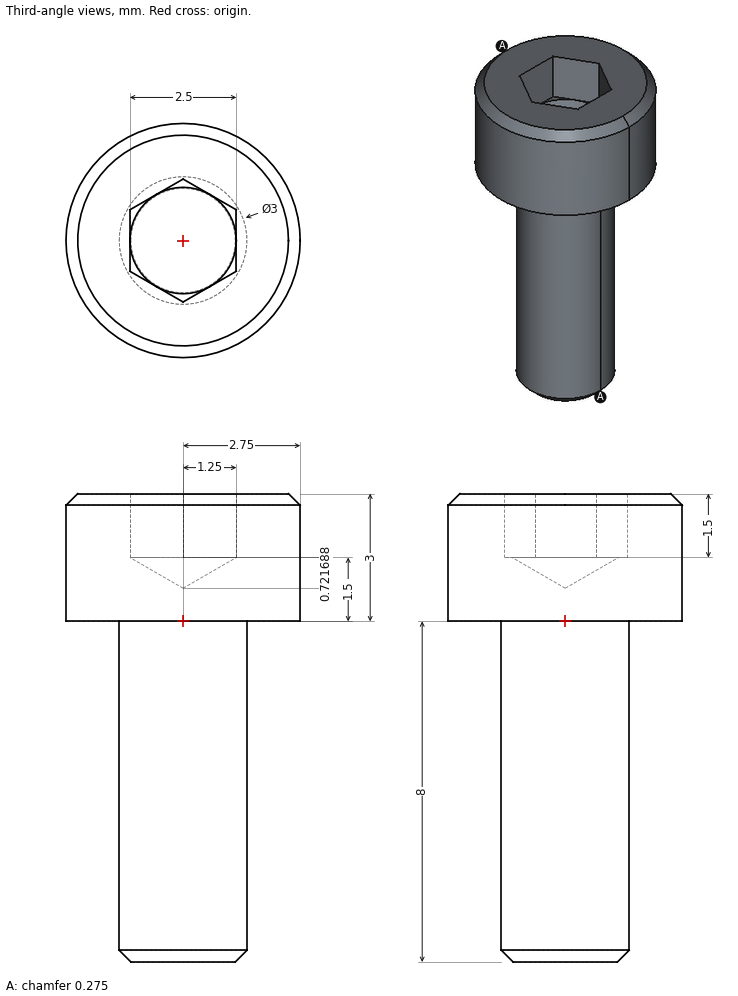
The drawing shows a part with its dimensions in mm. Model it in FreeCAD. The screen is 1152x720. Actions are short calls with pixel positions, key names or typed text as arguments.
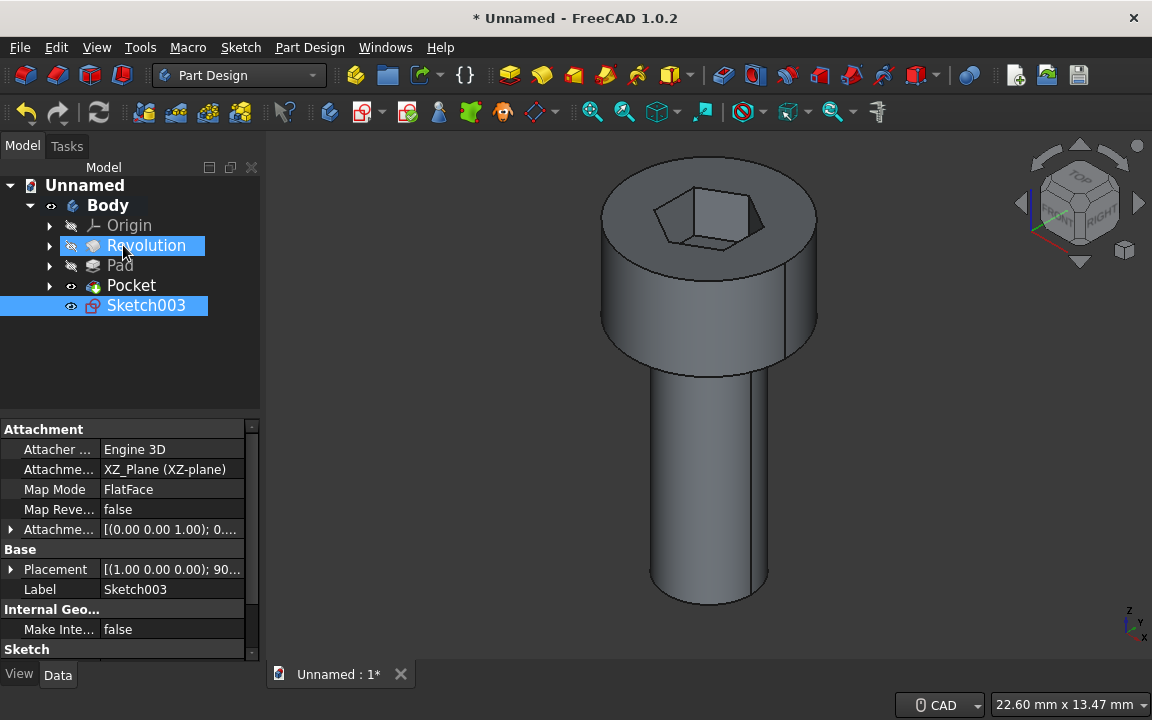
click(788, 76)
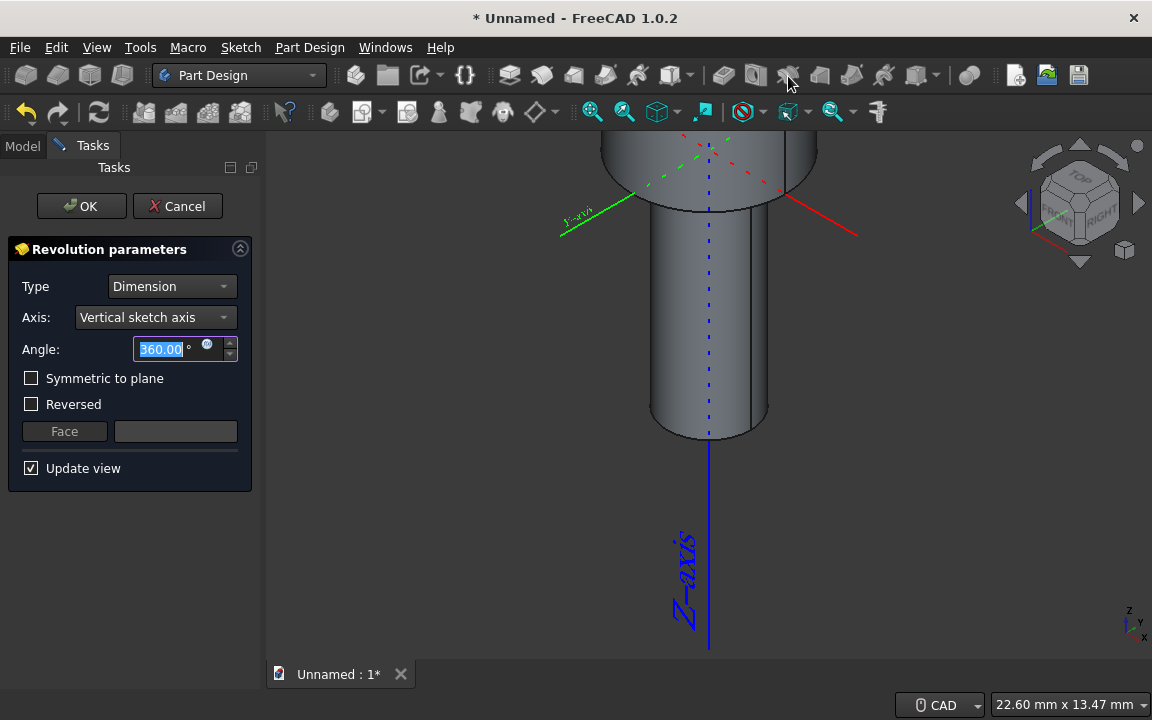
click(82, 206)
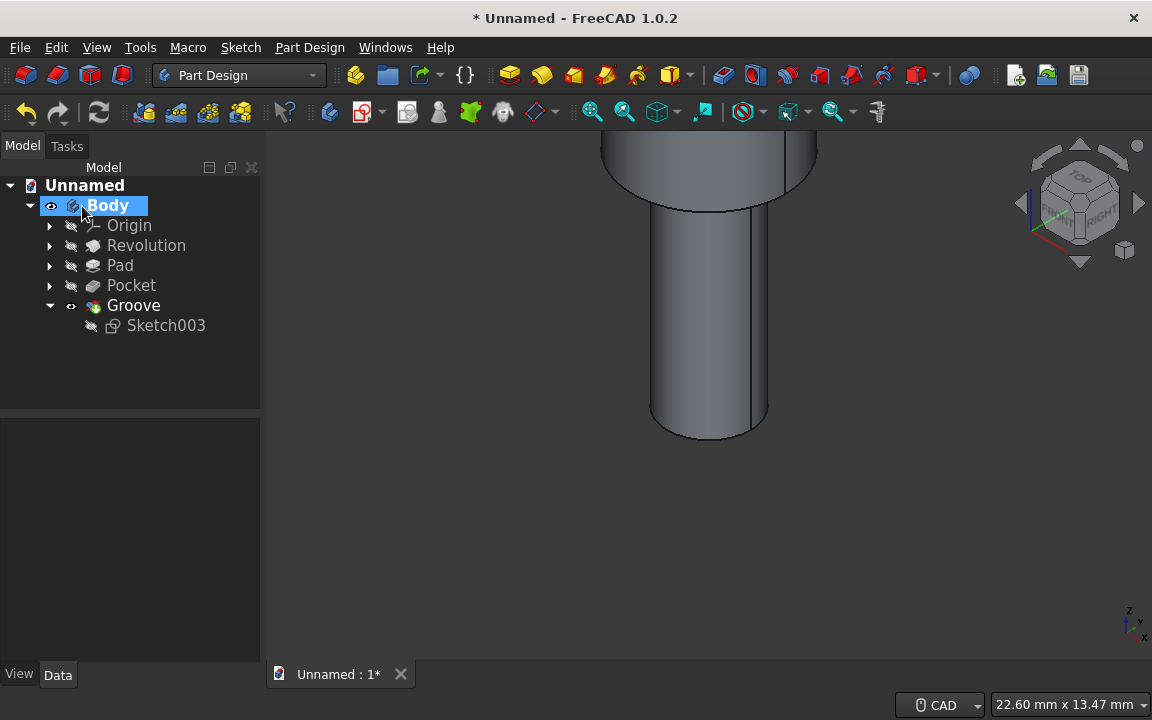
click(594, 112)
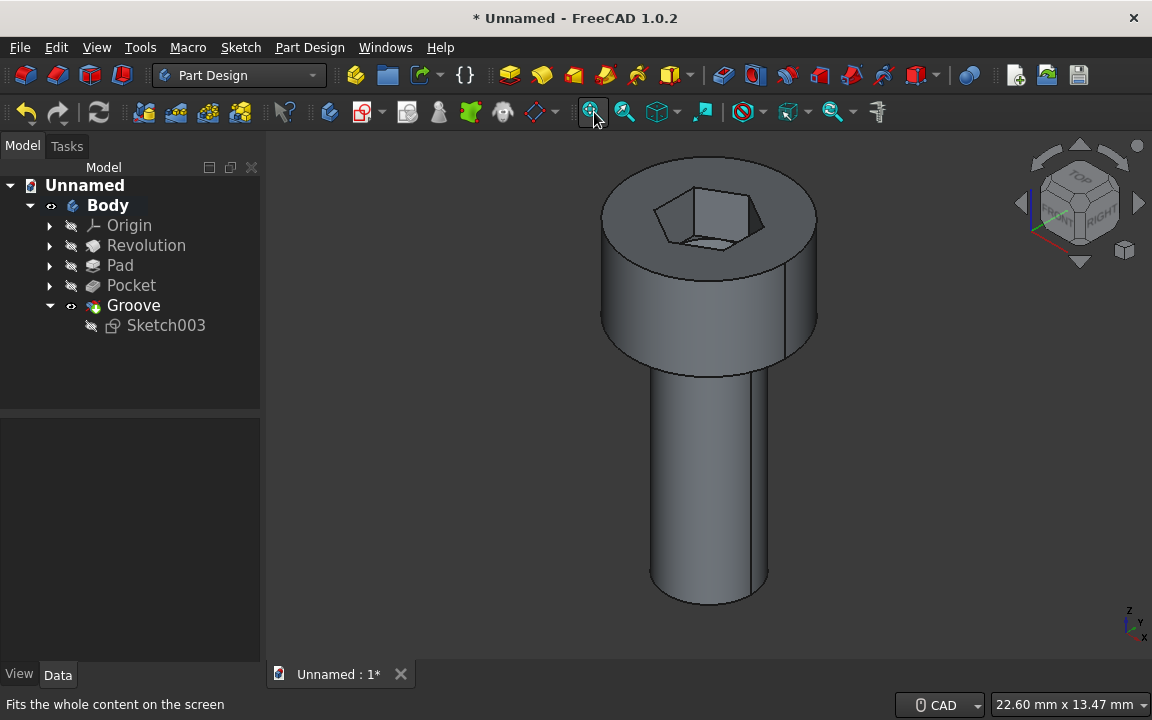
click(613, 246)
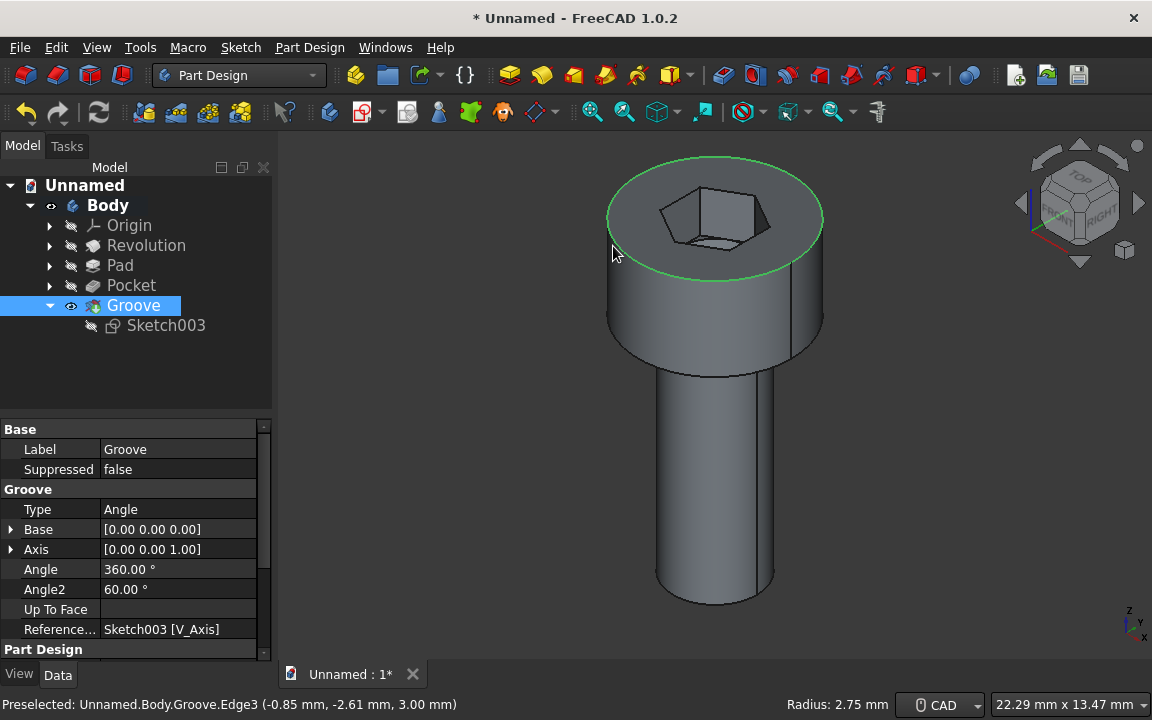
key(2)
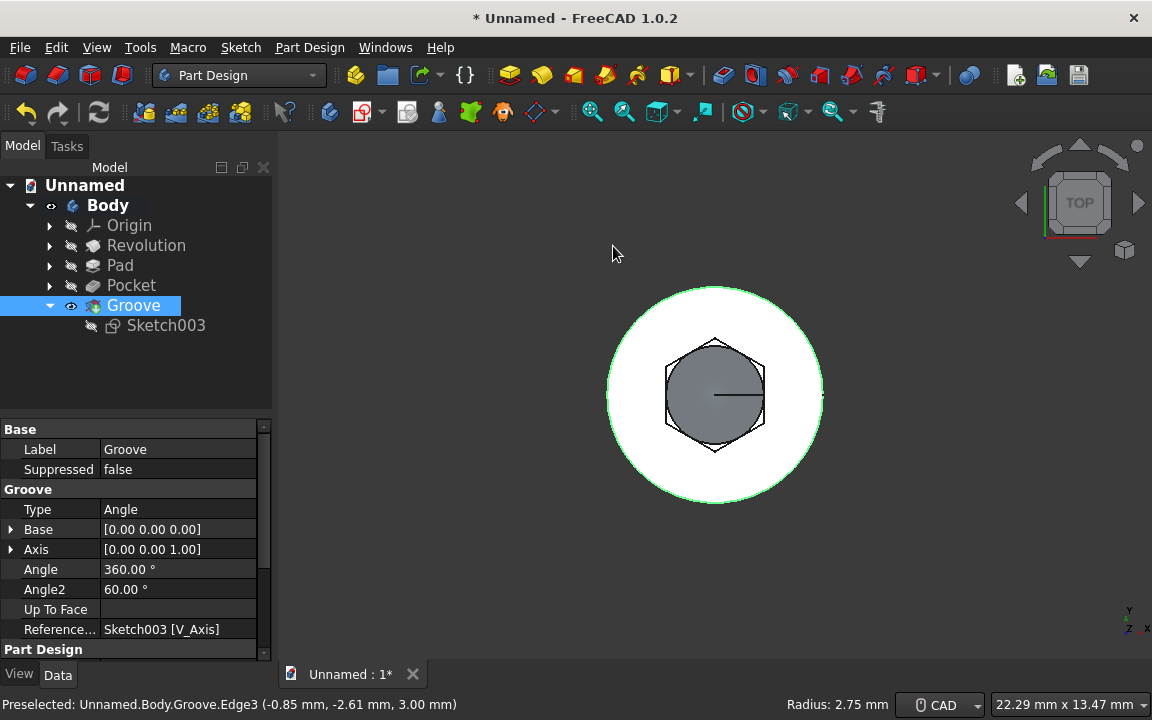
key(v)
key(f)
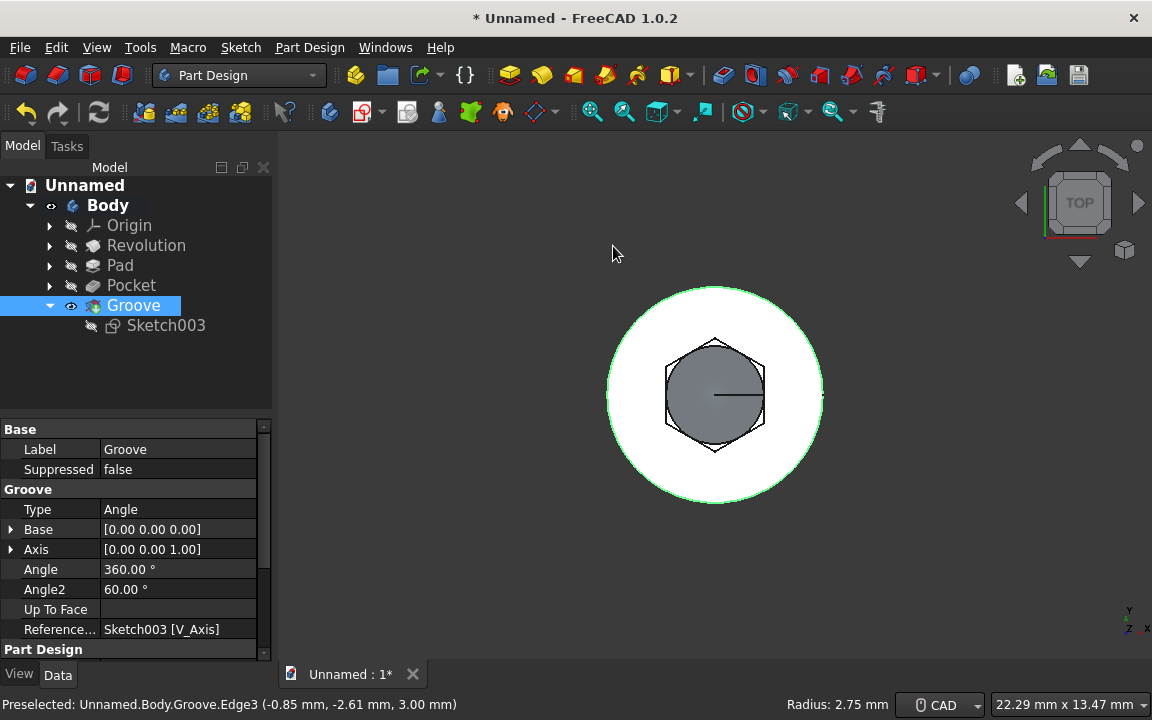
key(0)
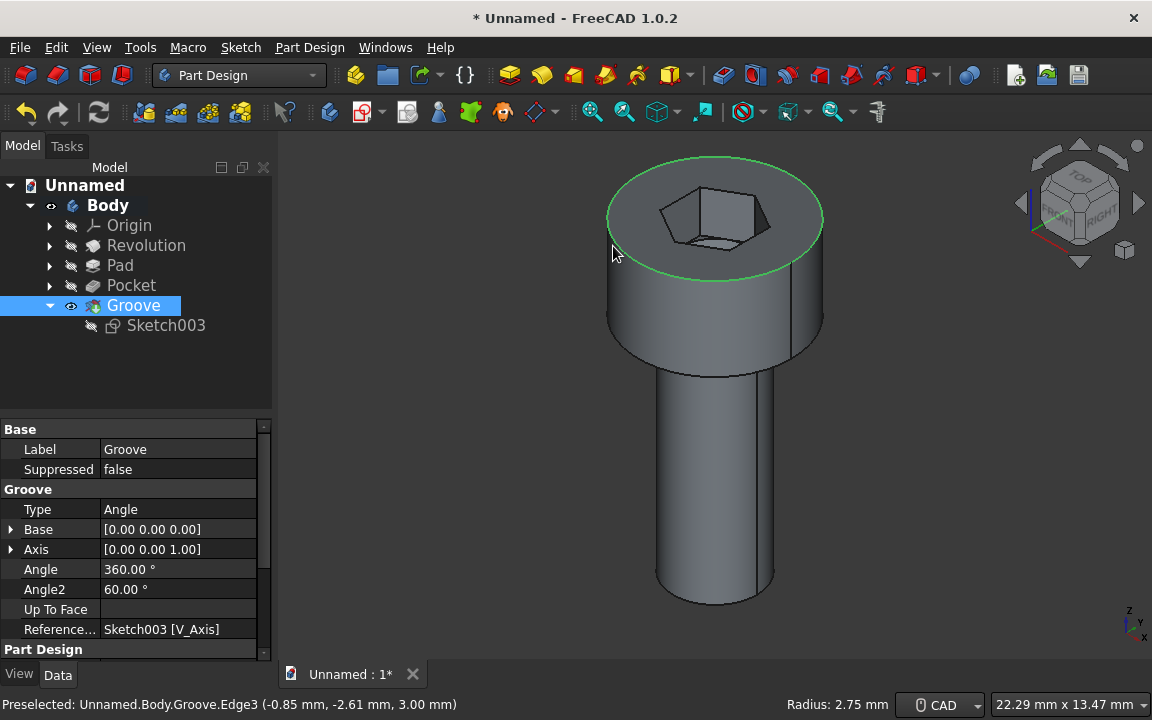
click(594, 112)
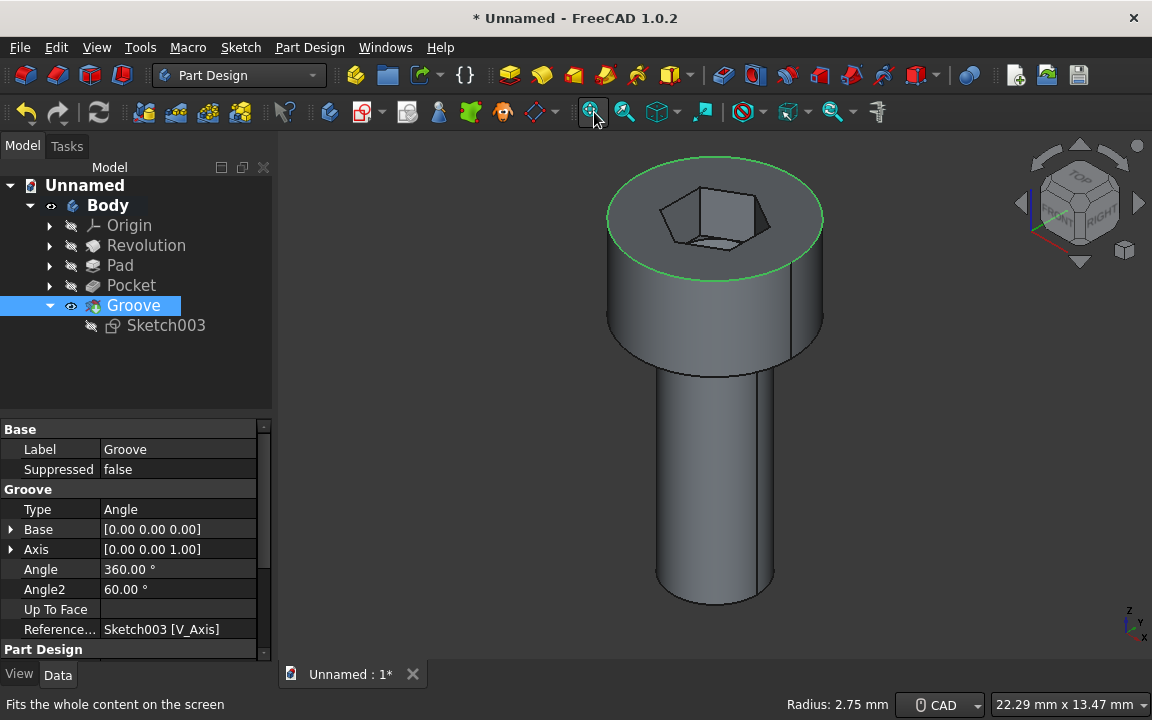
key(1)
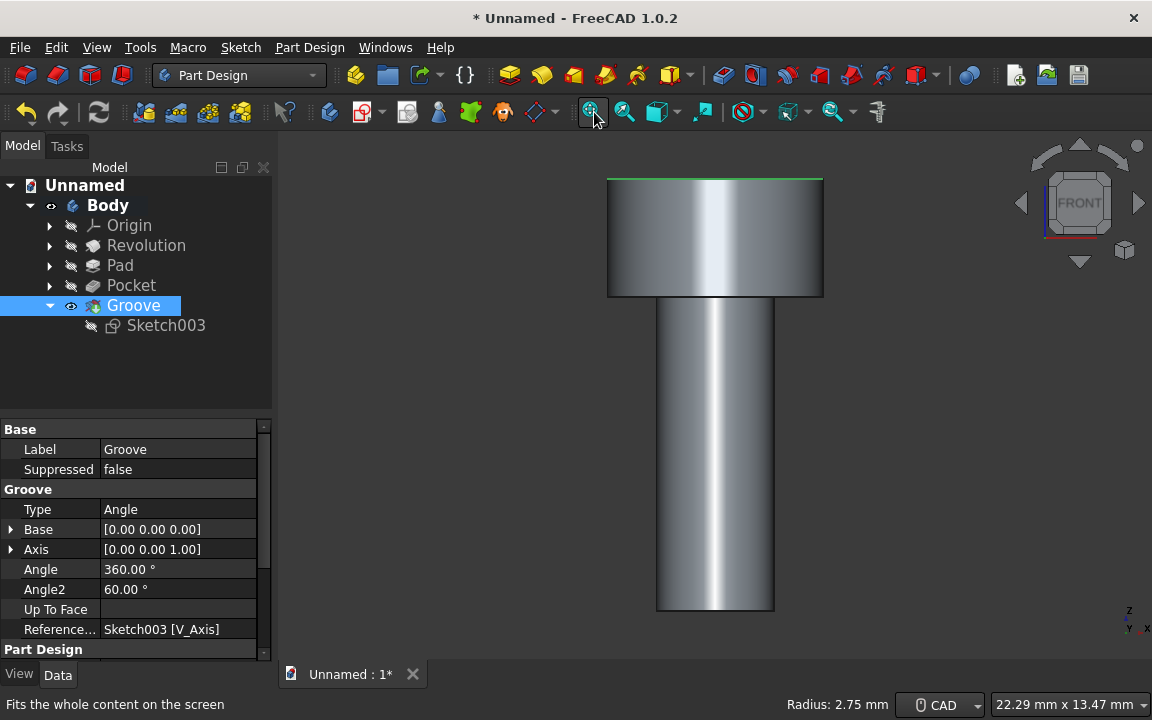
click(758, 610, ctrl)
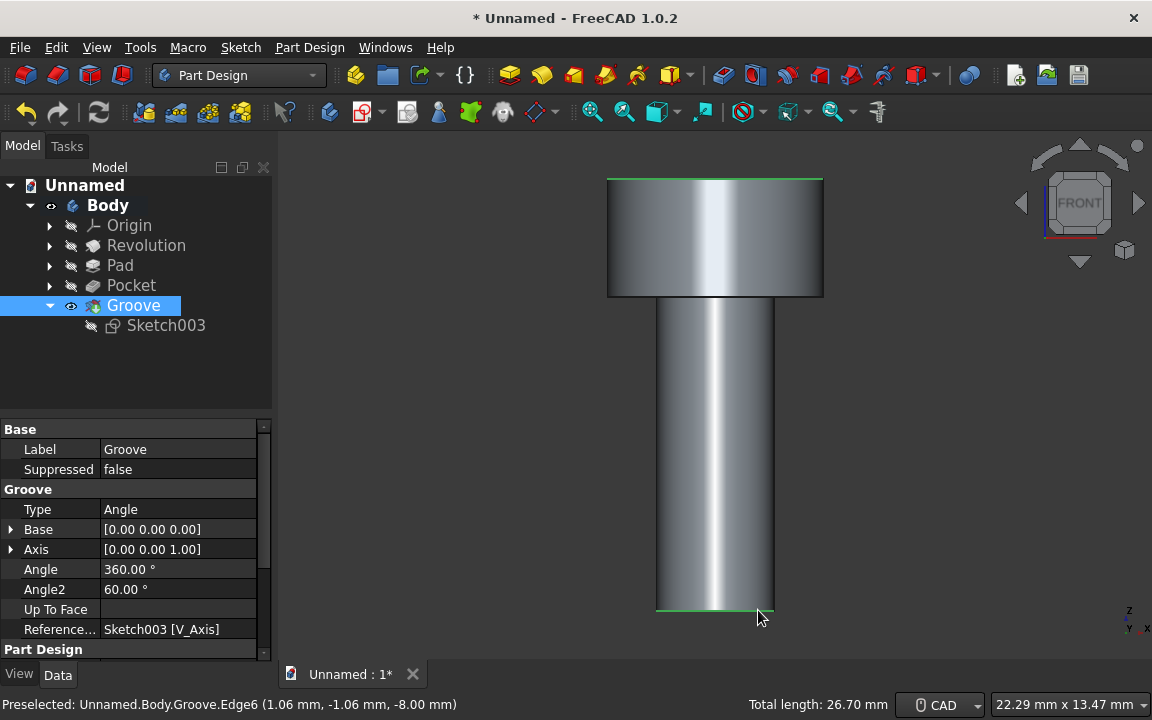
click(58, 76)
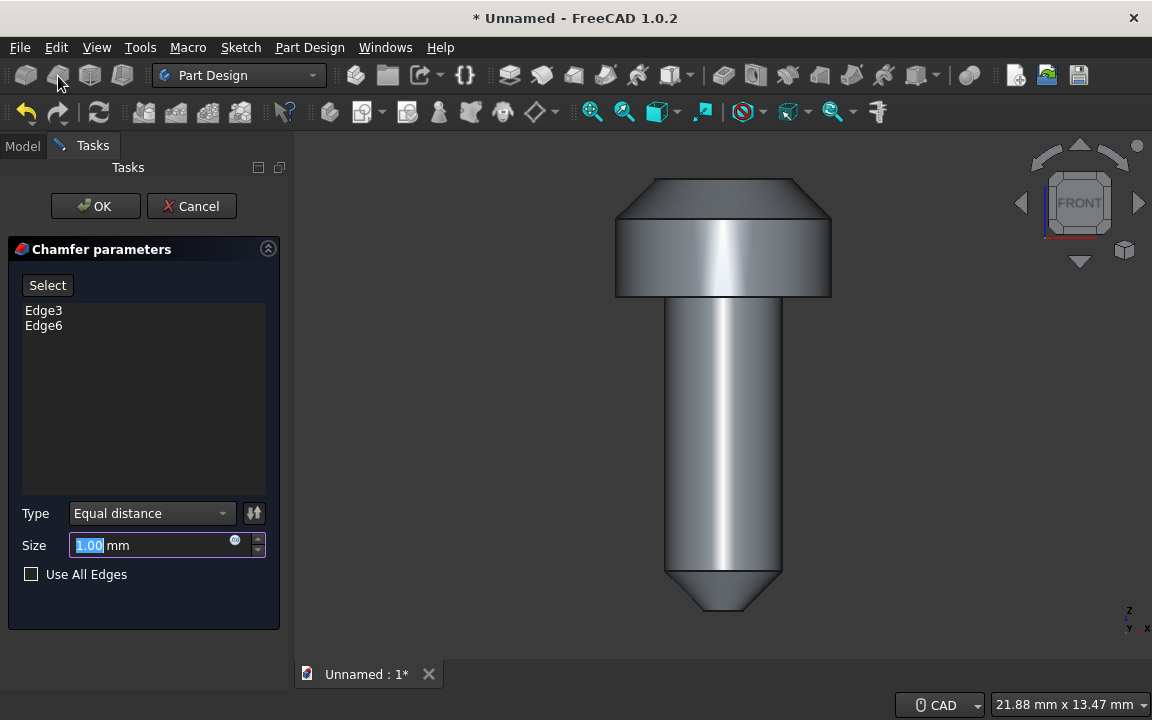
text(0.275)
key(Tab)